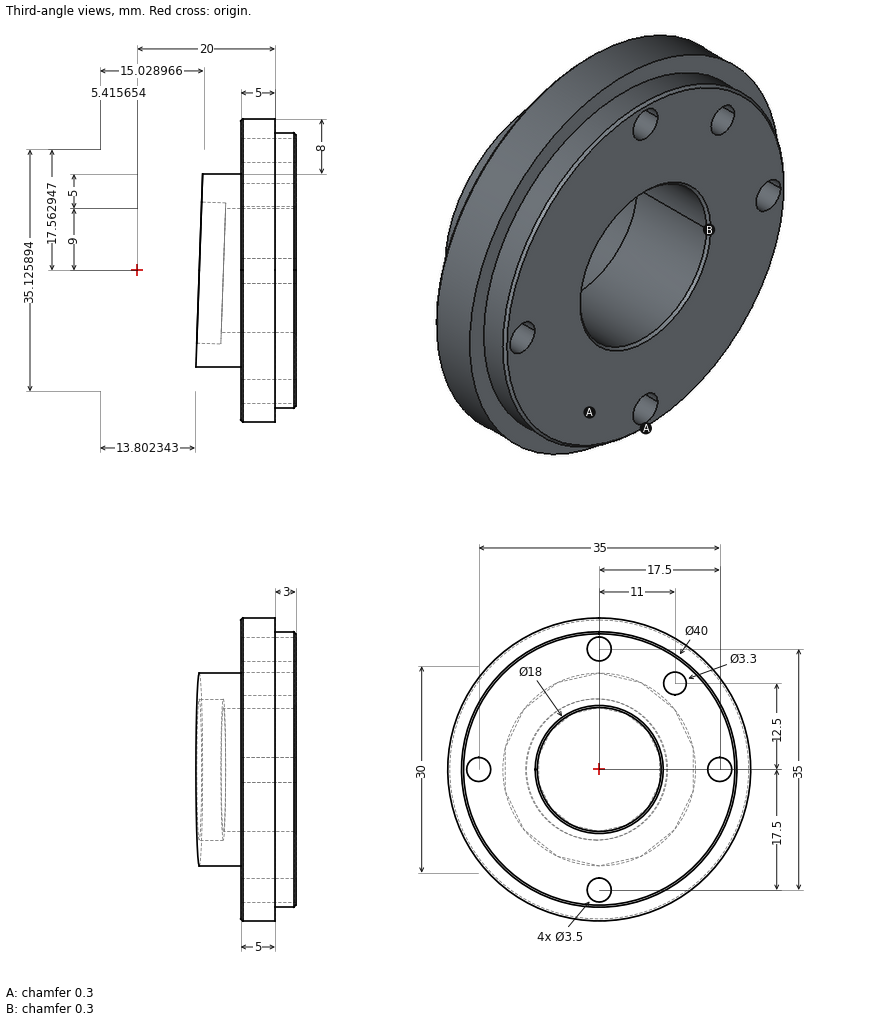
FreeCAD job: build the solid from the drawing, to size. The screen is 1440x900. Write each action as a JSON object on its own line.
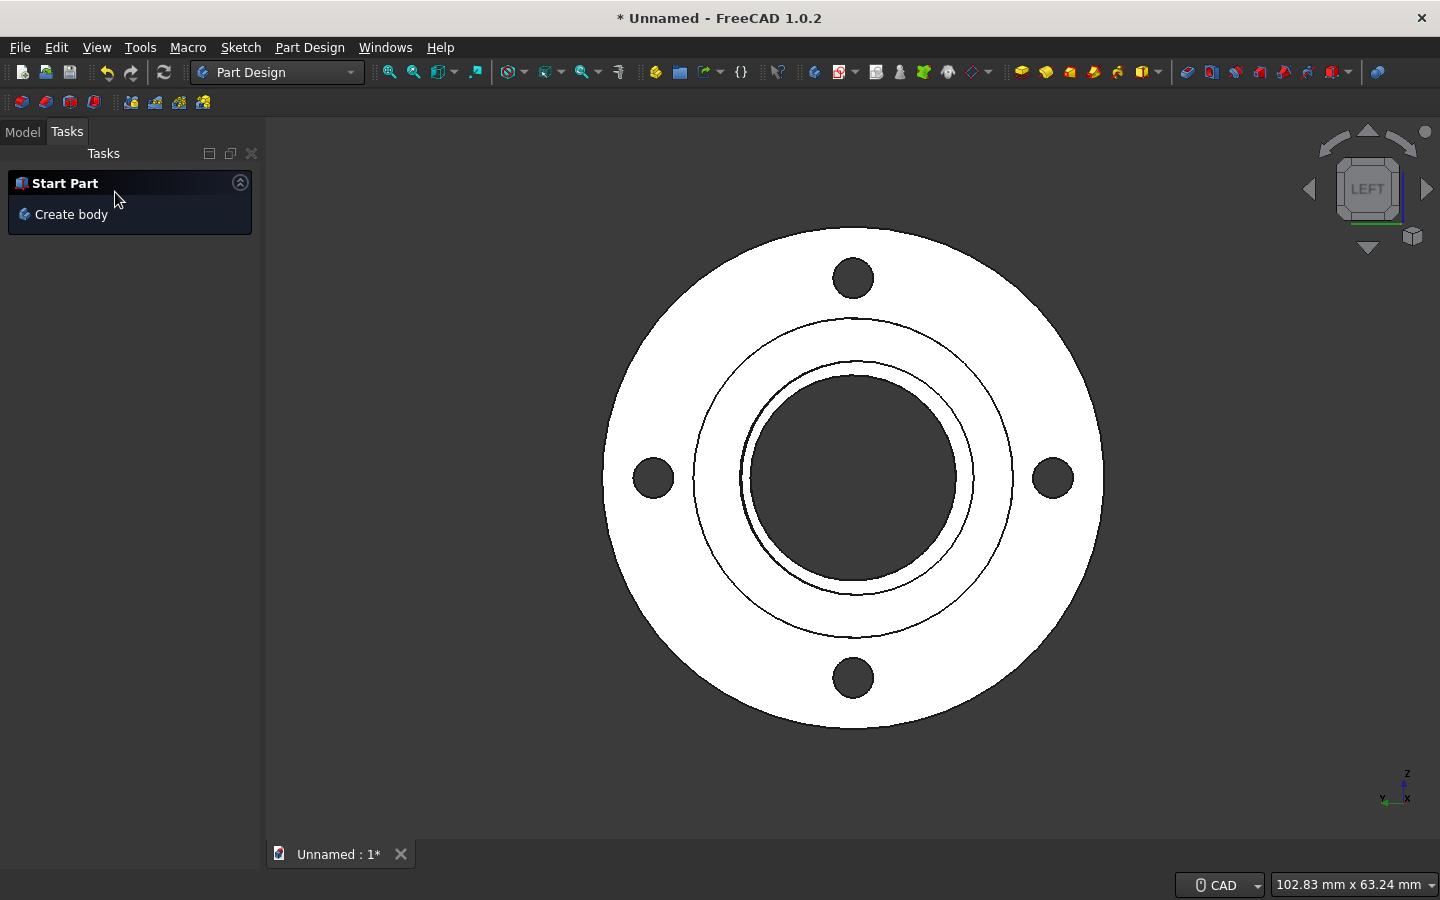
{"action": "key", "text": "0"}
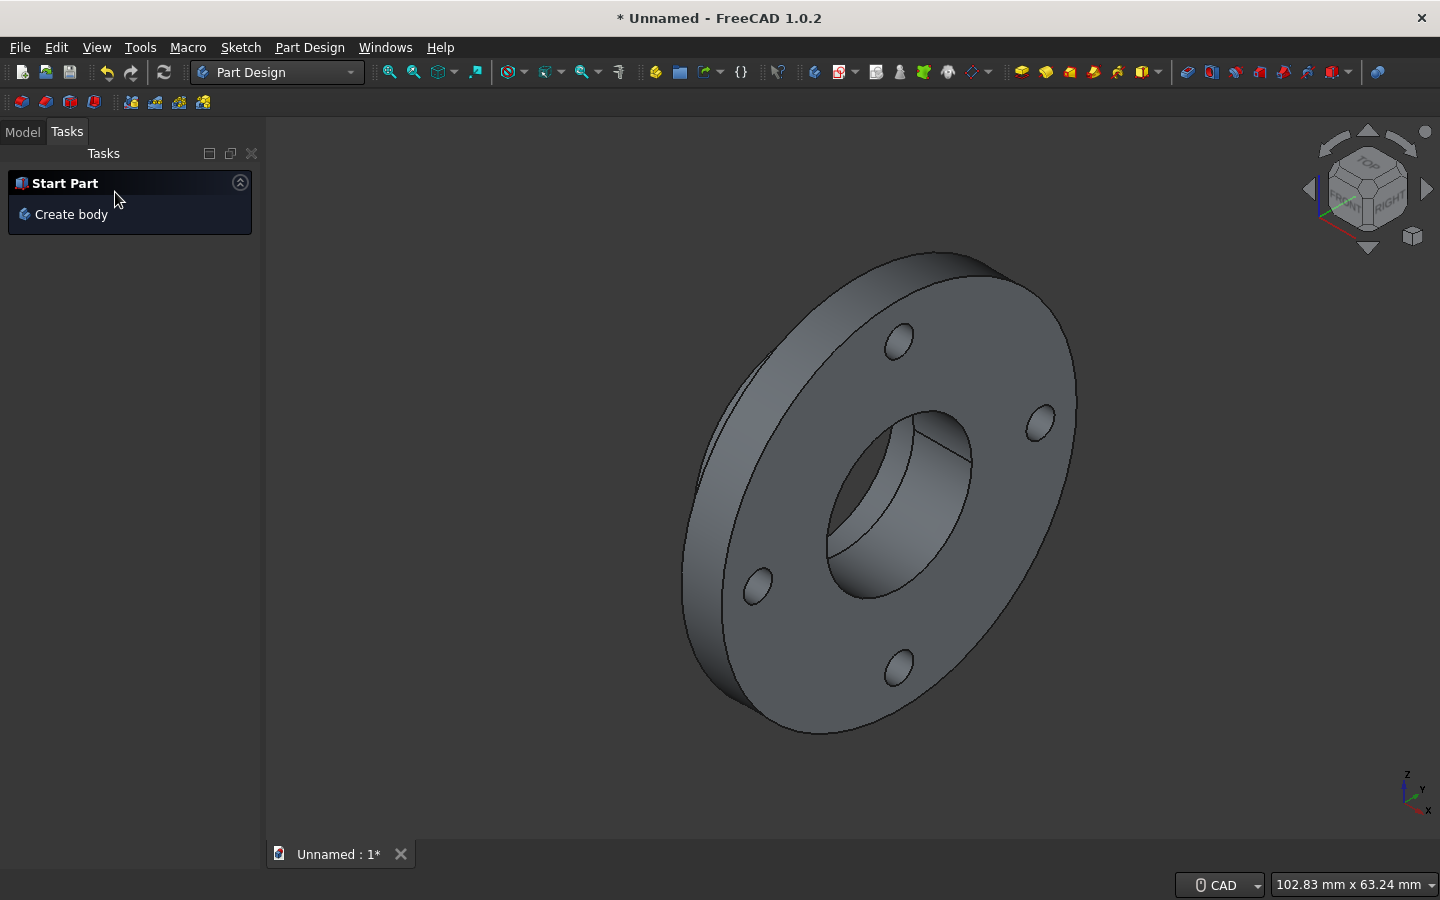
{"action": "left_click", "coordinate": [1001, 387]}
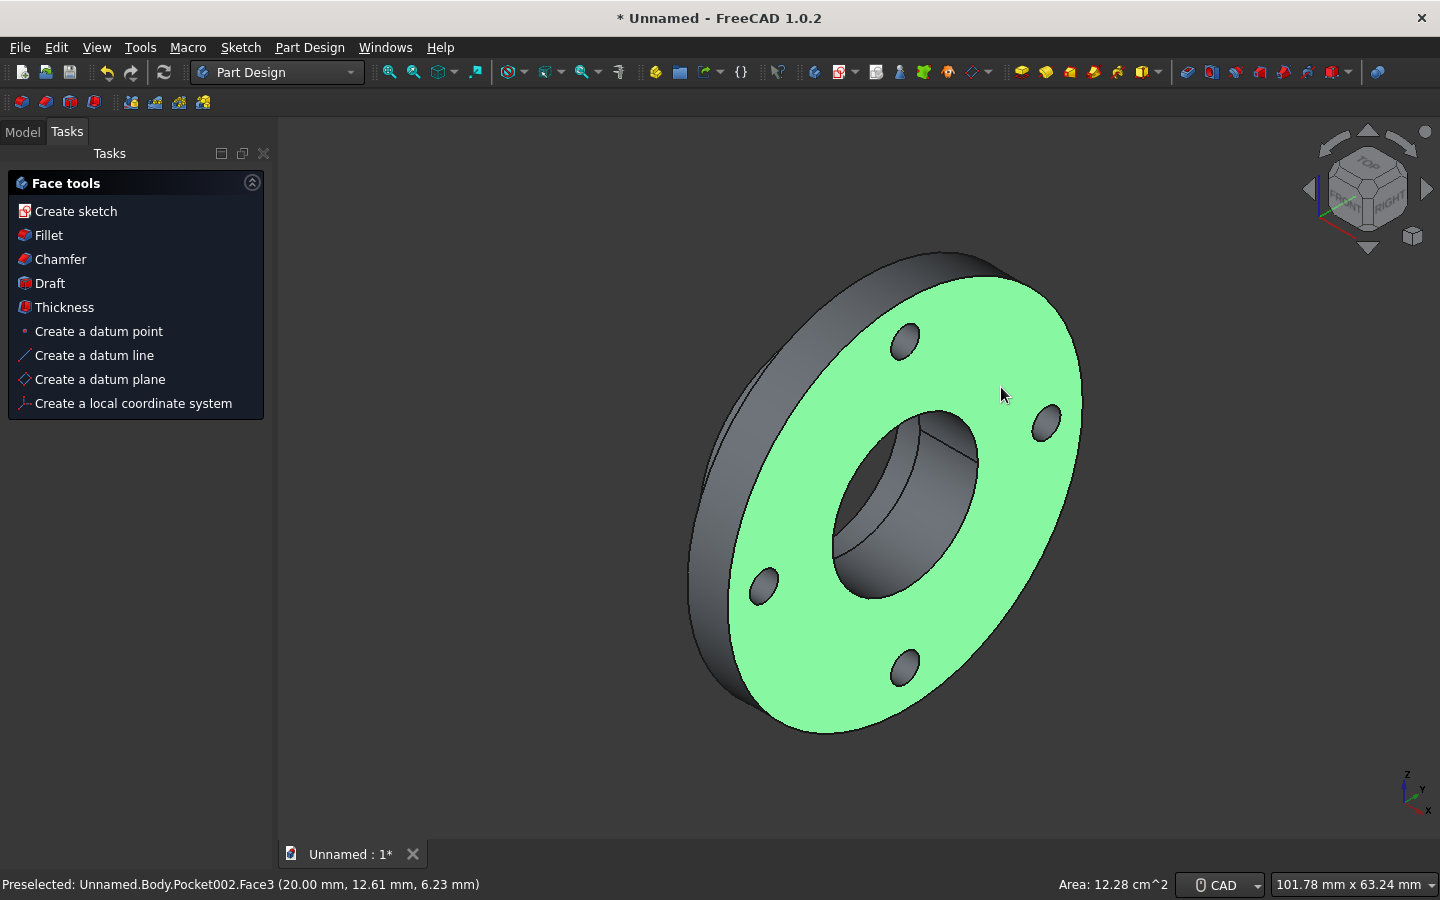
{"action": "left_click", "coordinate": [840, 72]}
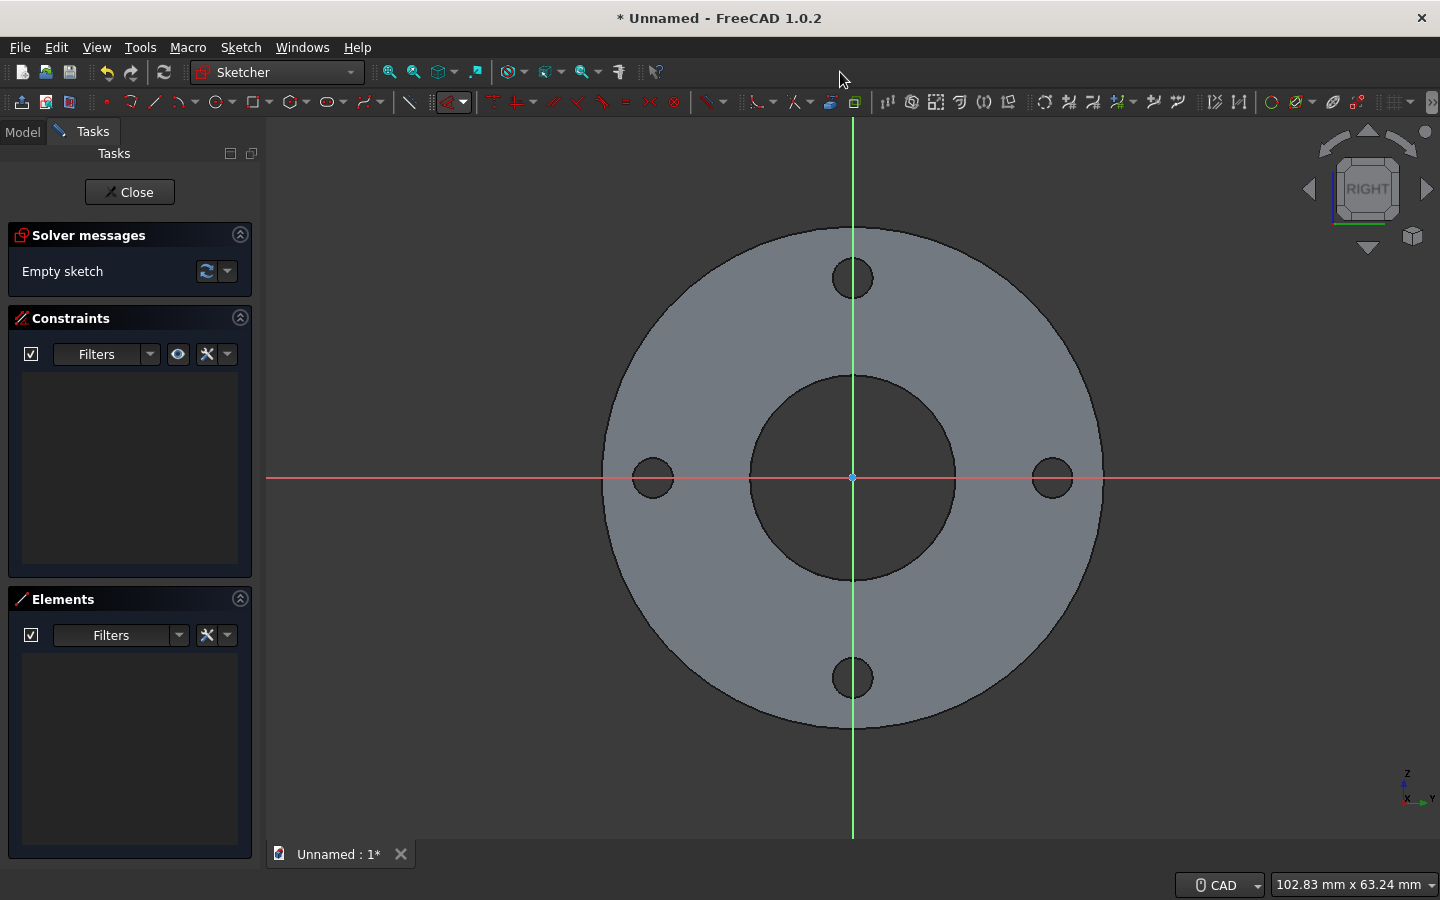
{"action": "key", "text": "g c"}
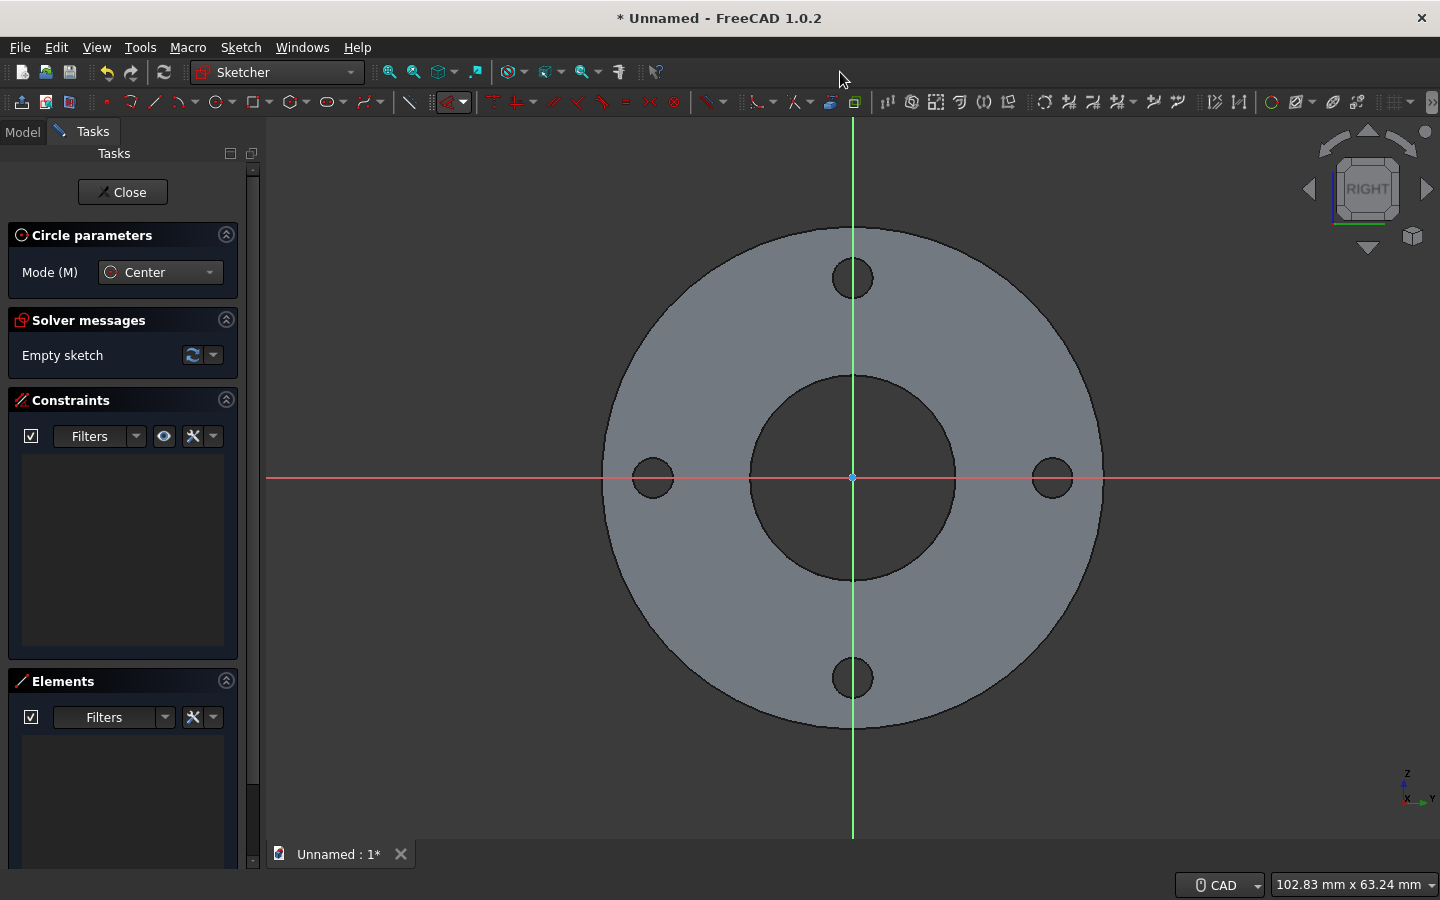
{"action": "left_click", "coordinate": [853, 478]}
{"action": "mouse_move", "coordinate": [1014, 317]}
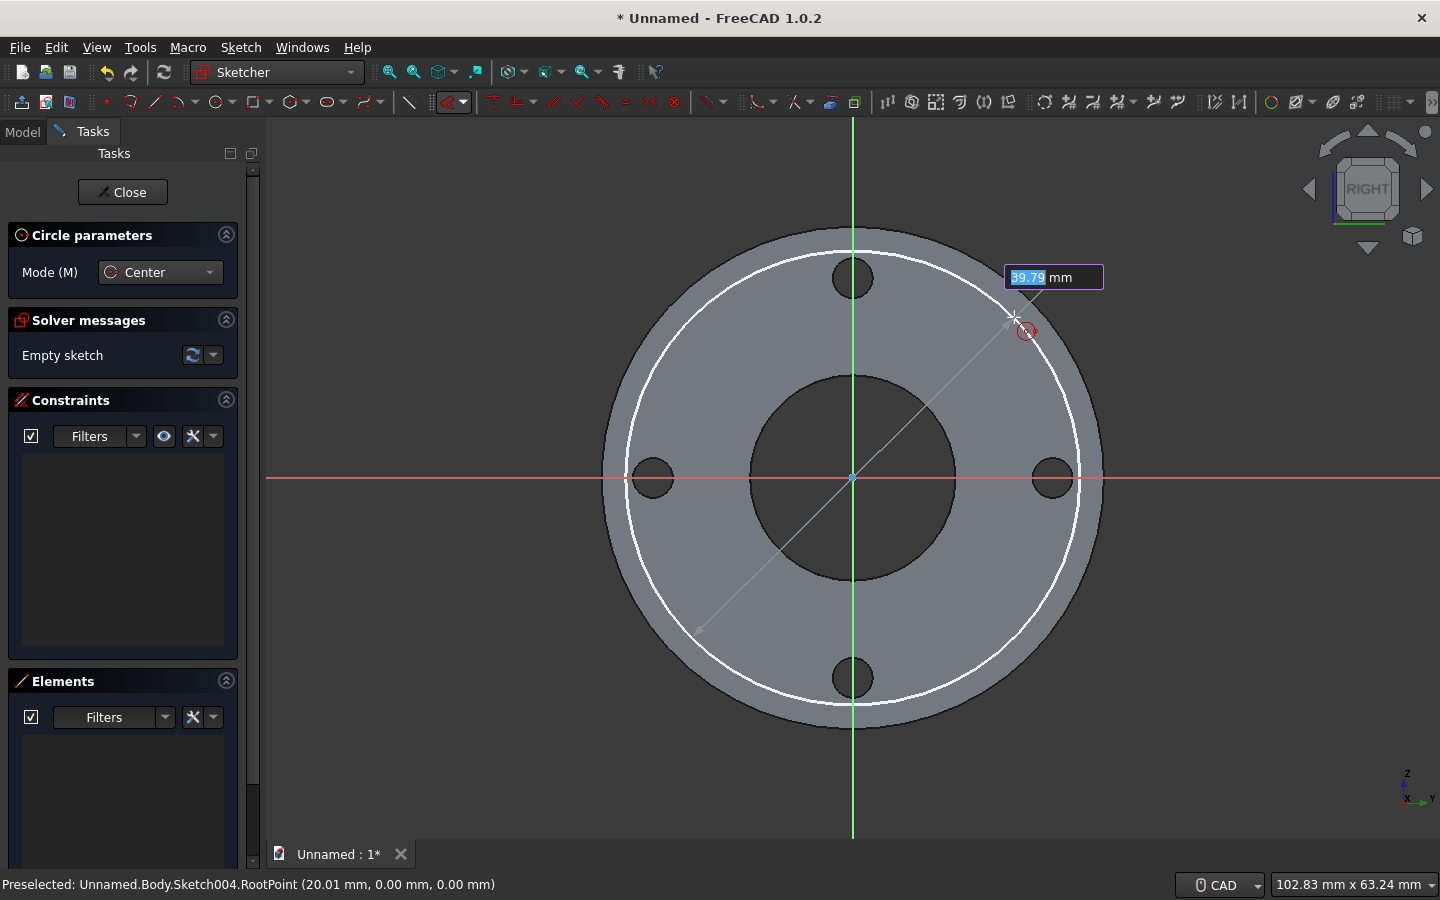
{"action": "type", "text": "40"}
{"action": "key", "text": "Return"}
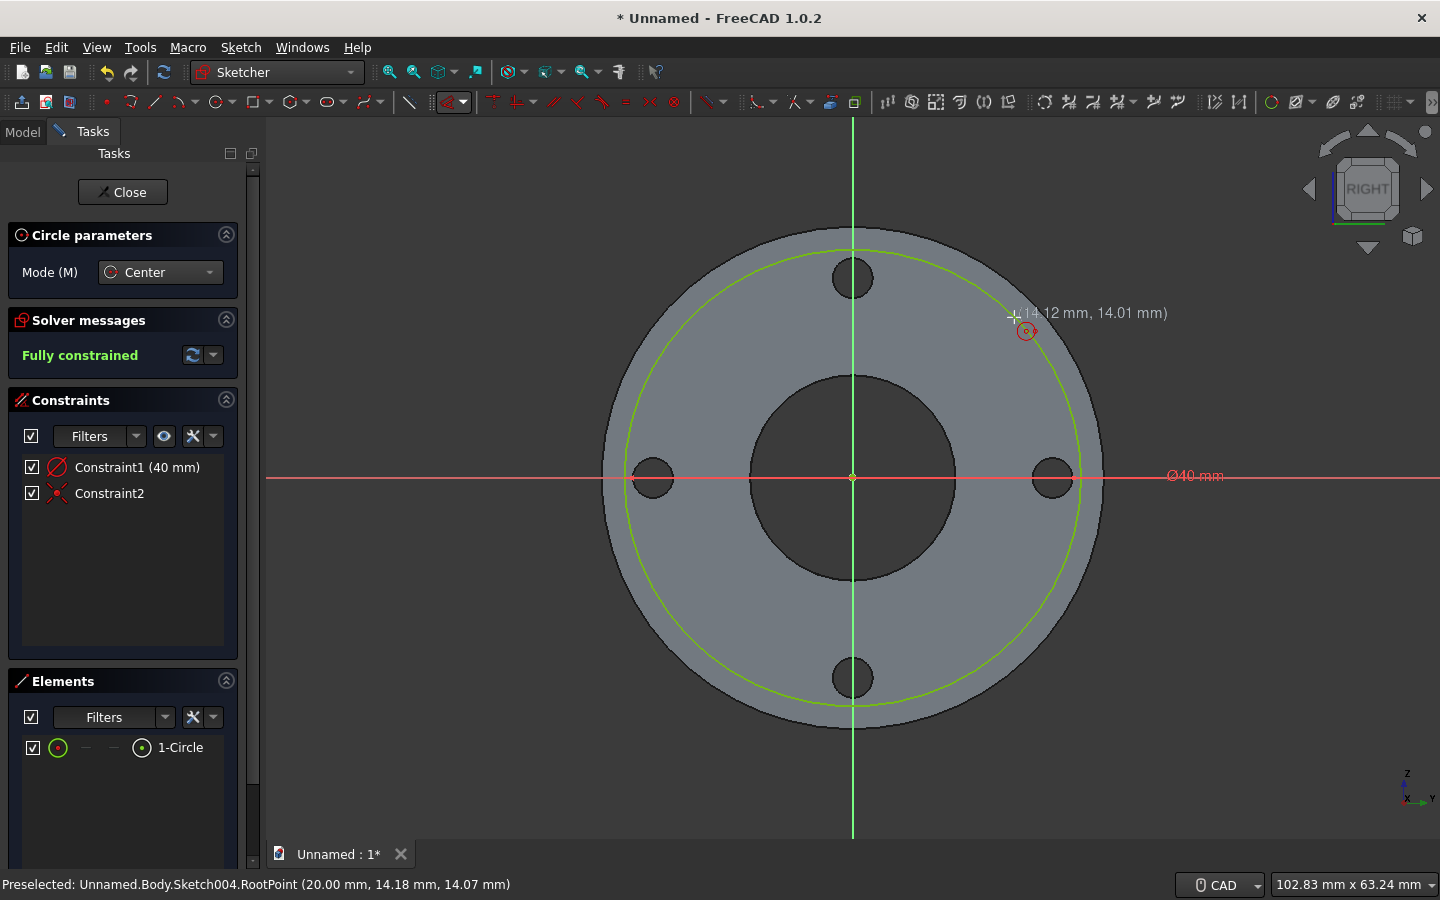
{"action": "left_click", "coordinate": [853, 678]}
{"action": "mouse_move", "coordinate": [867, 664]}